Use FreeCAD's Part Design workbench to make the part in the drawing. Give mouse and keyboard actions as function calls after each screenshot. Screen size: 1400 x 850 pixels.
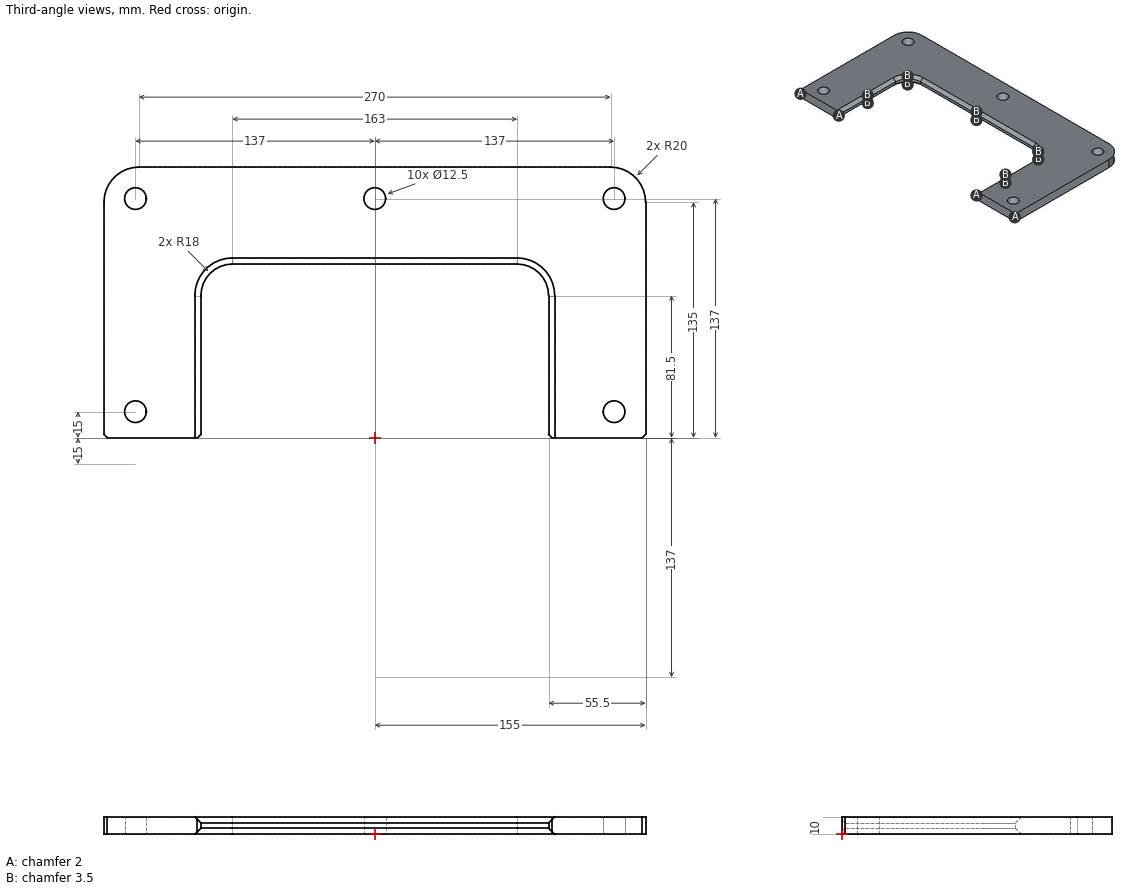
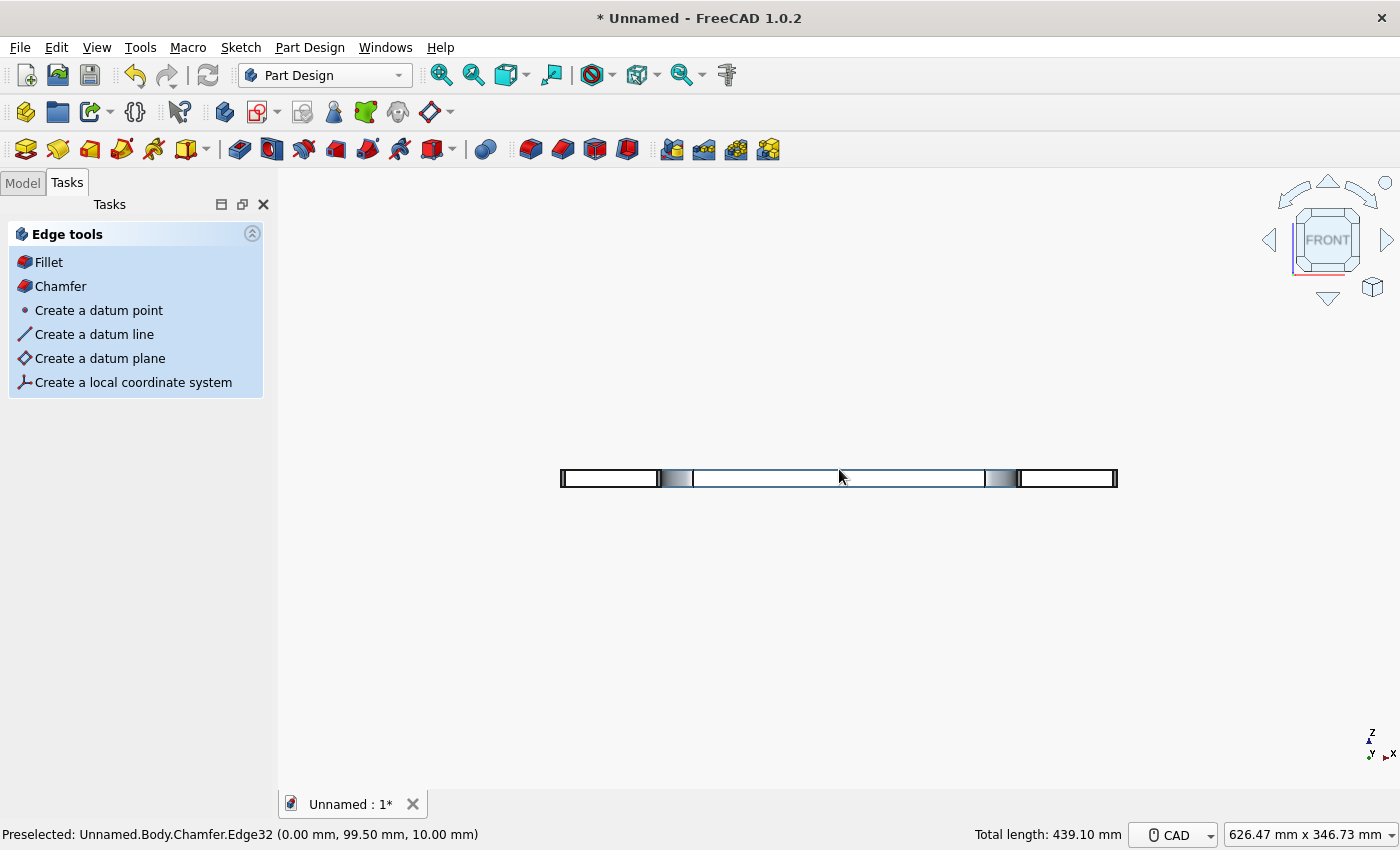
key(0)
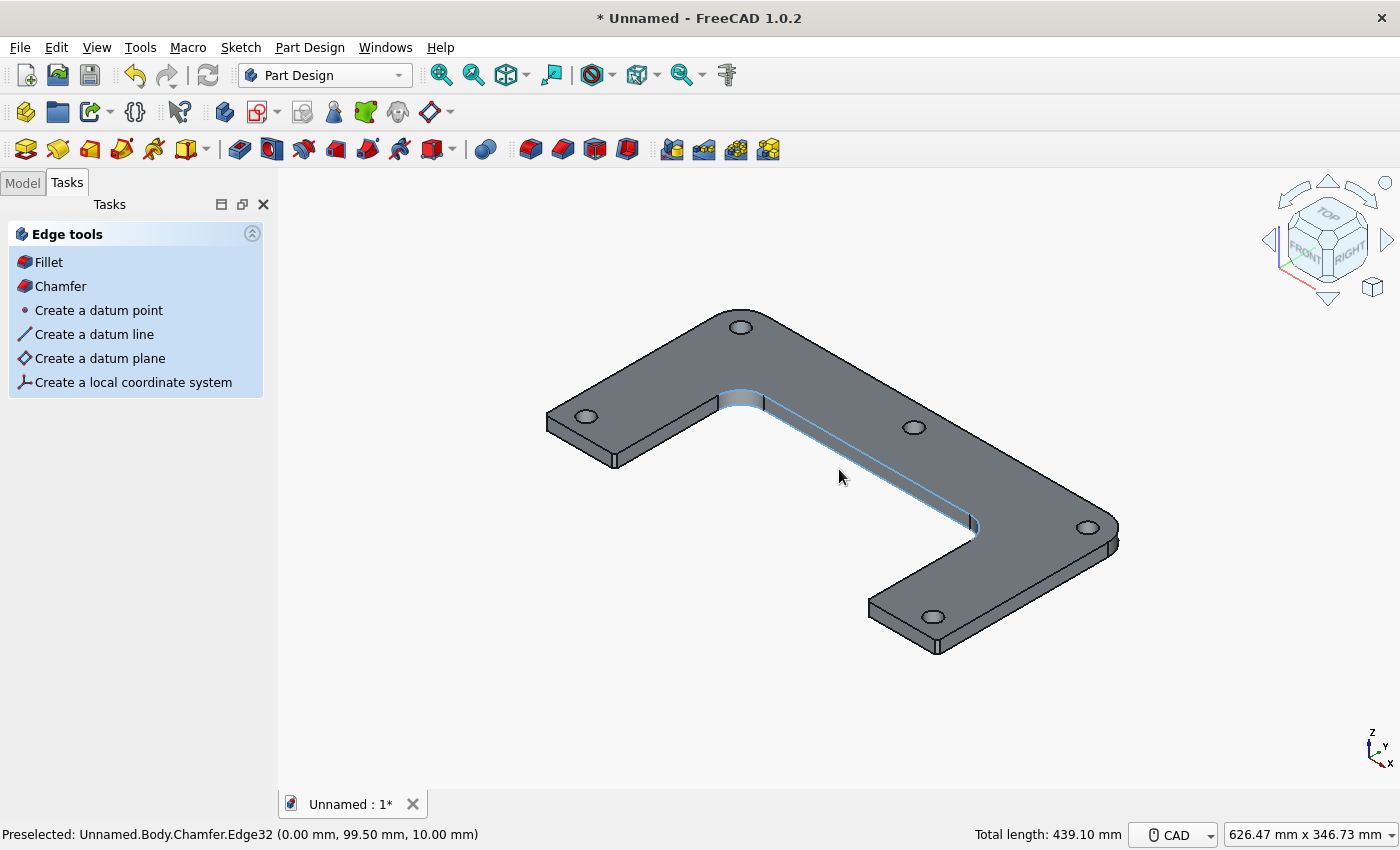
click(668, 424, ctrl)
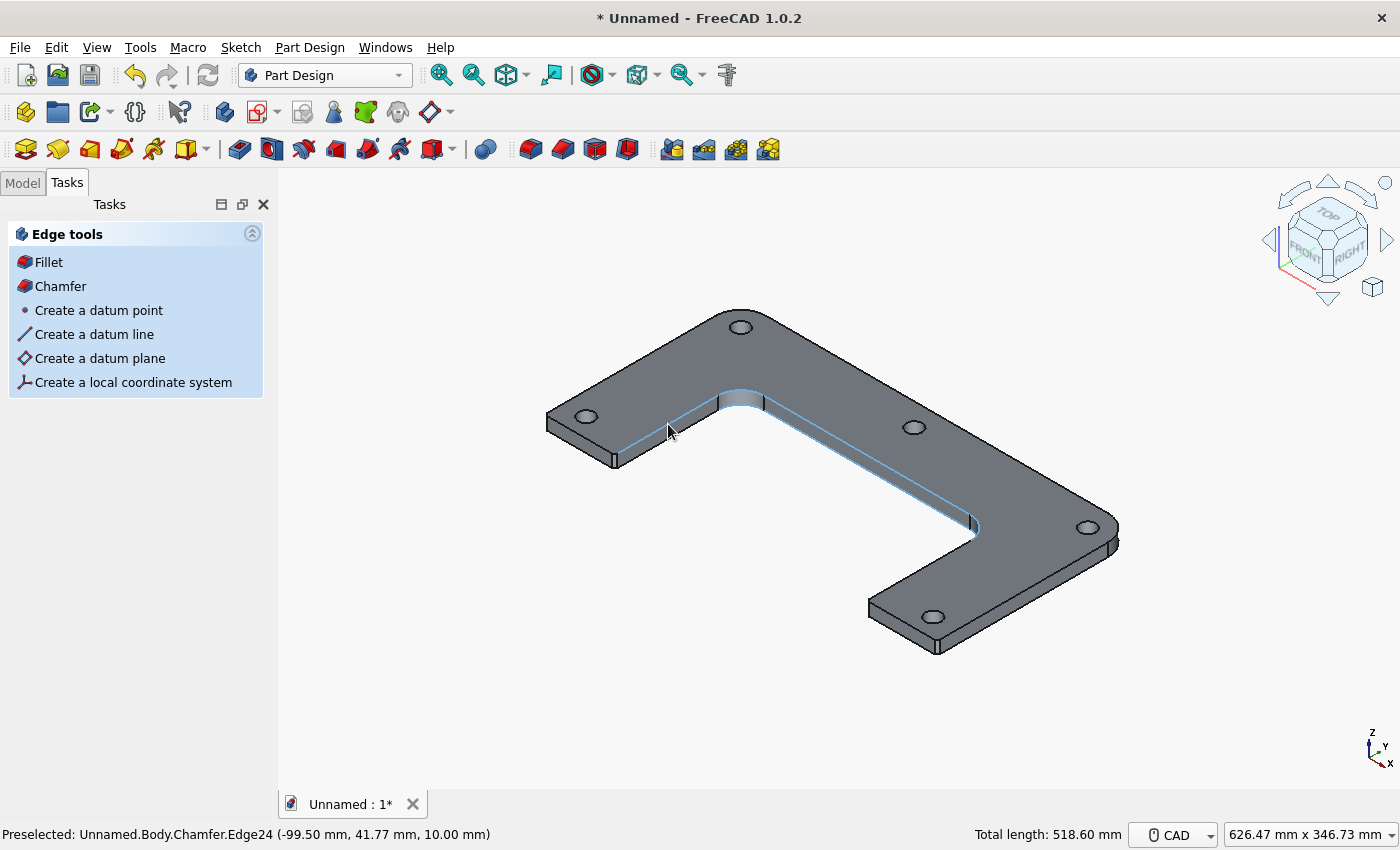
key(2)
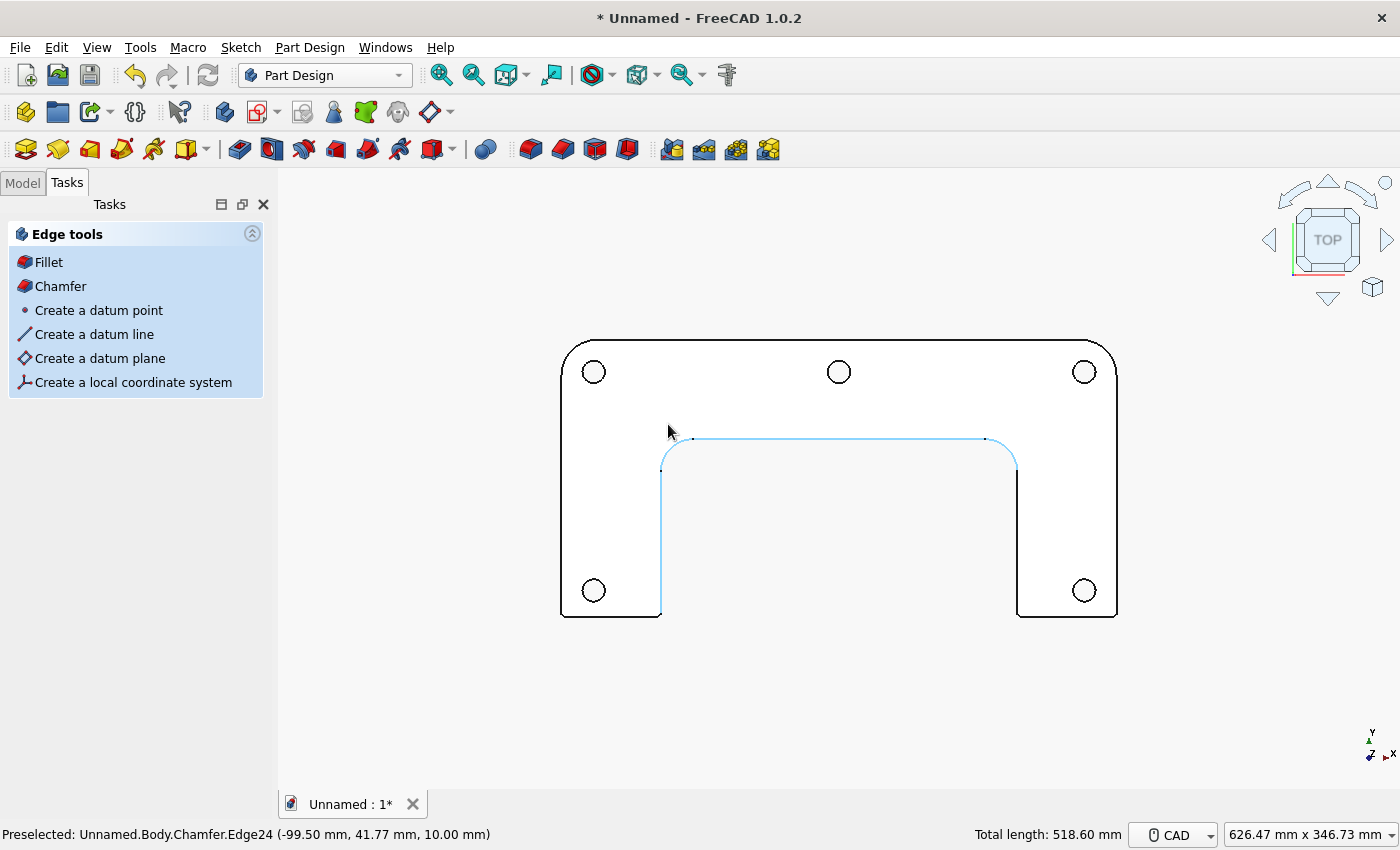
click(1017, 542, ctrl)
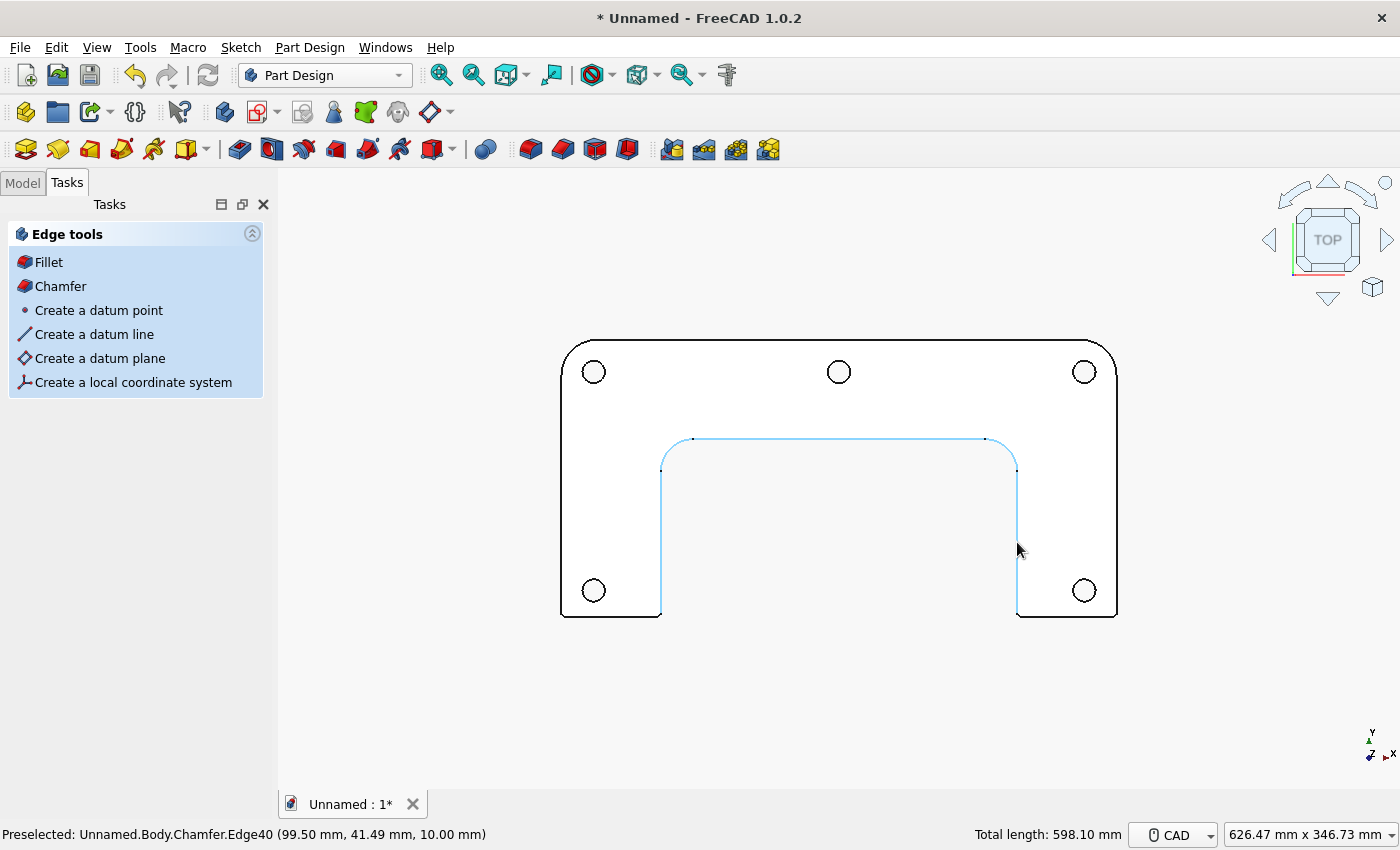
key(1)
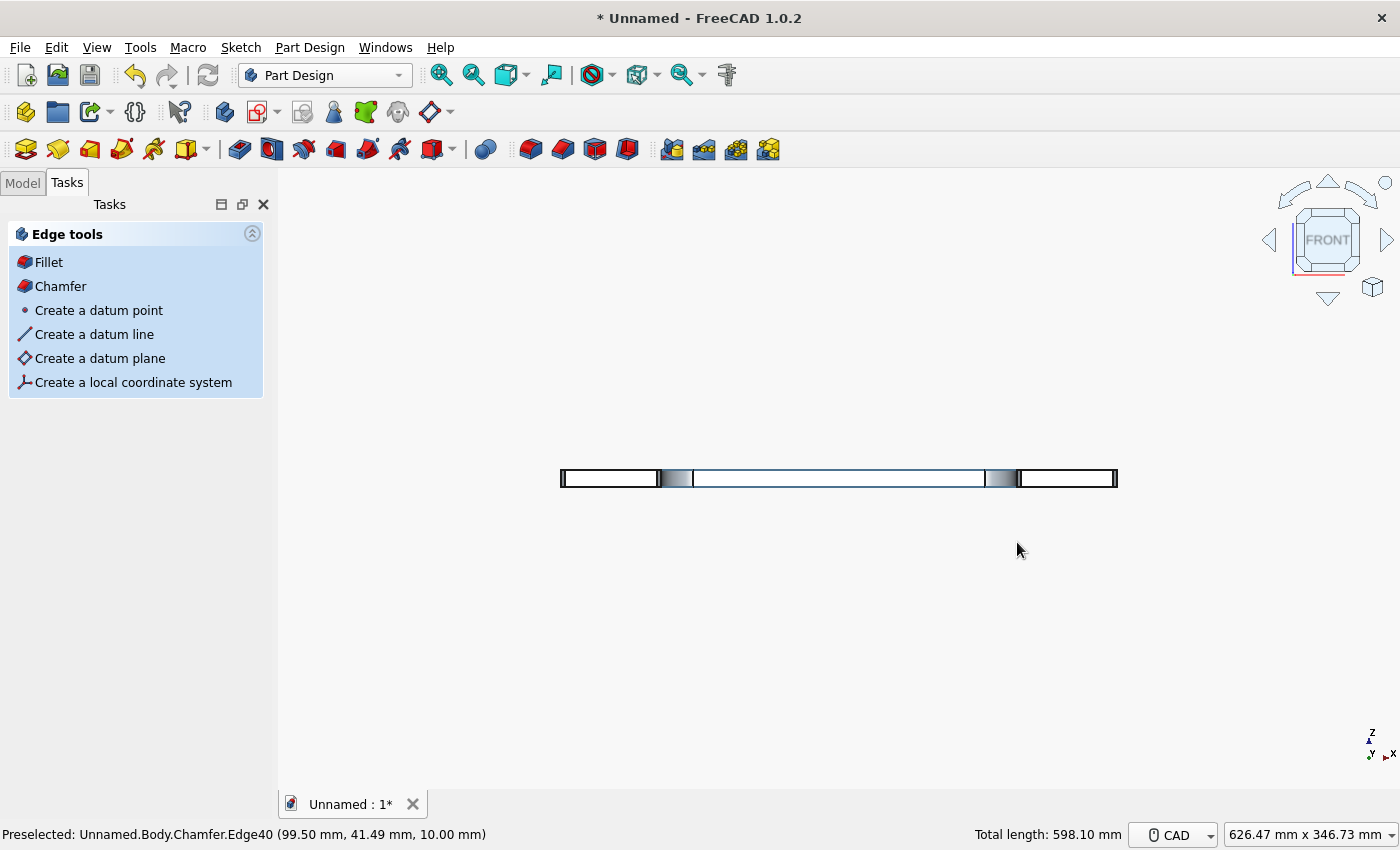
key(3)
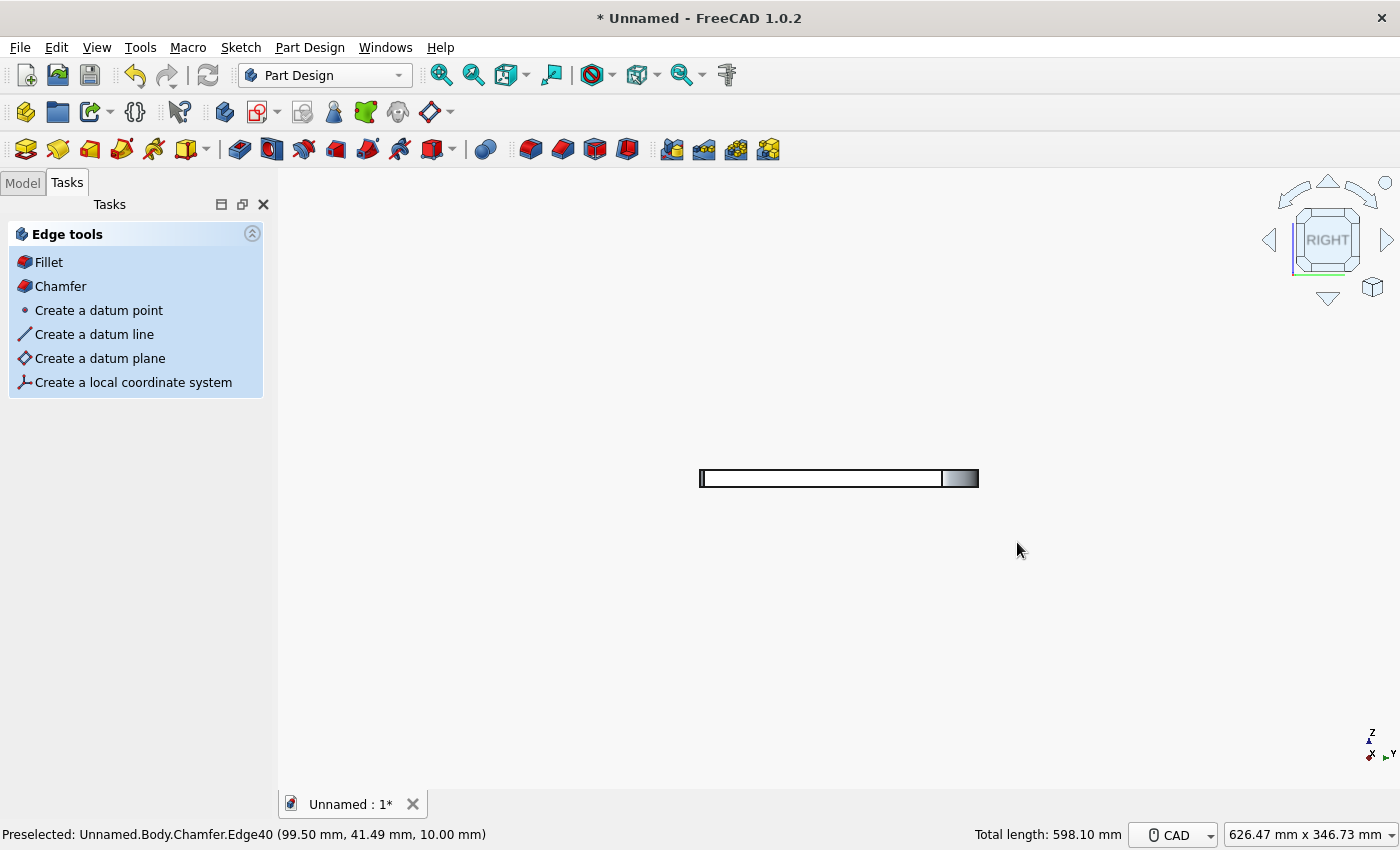
click(442, 76)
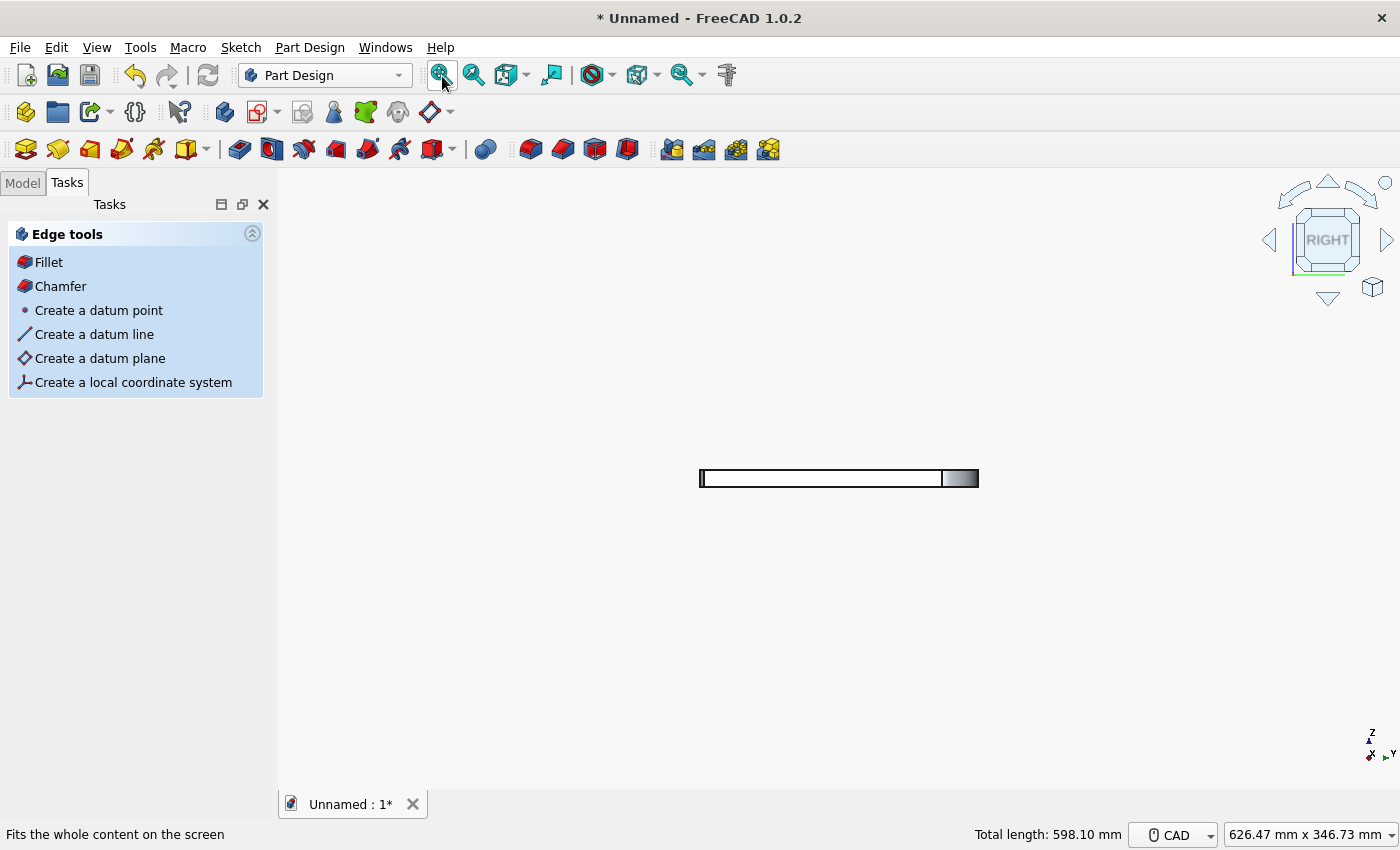
key(5)